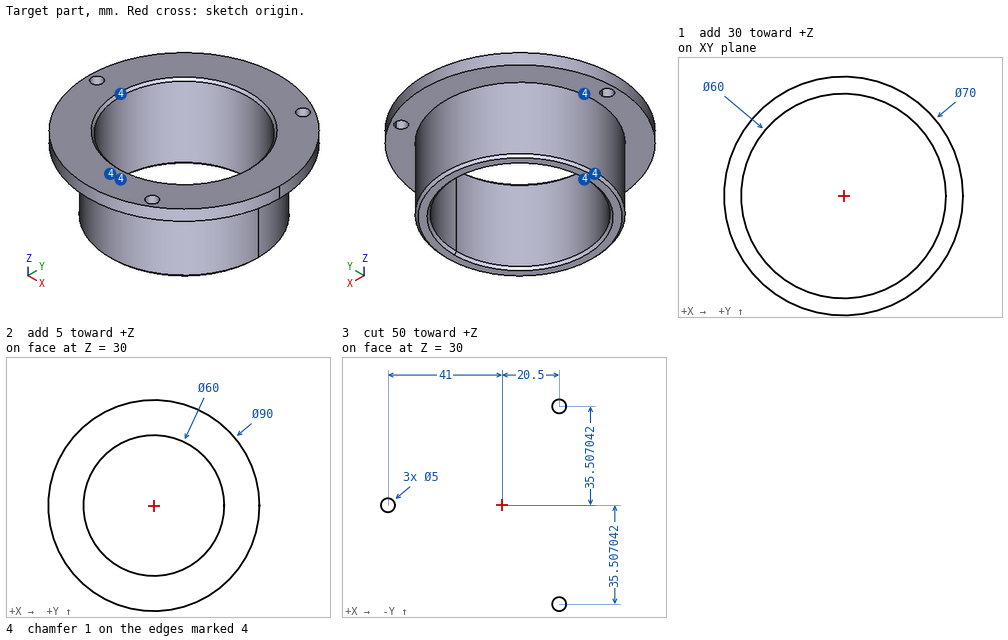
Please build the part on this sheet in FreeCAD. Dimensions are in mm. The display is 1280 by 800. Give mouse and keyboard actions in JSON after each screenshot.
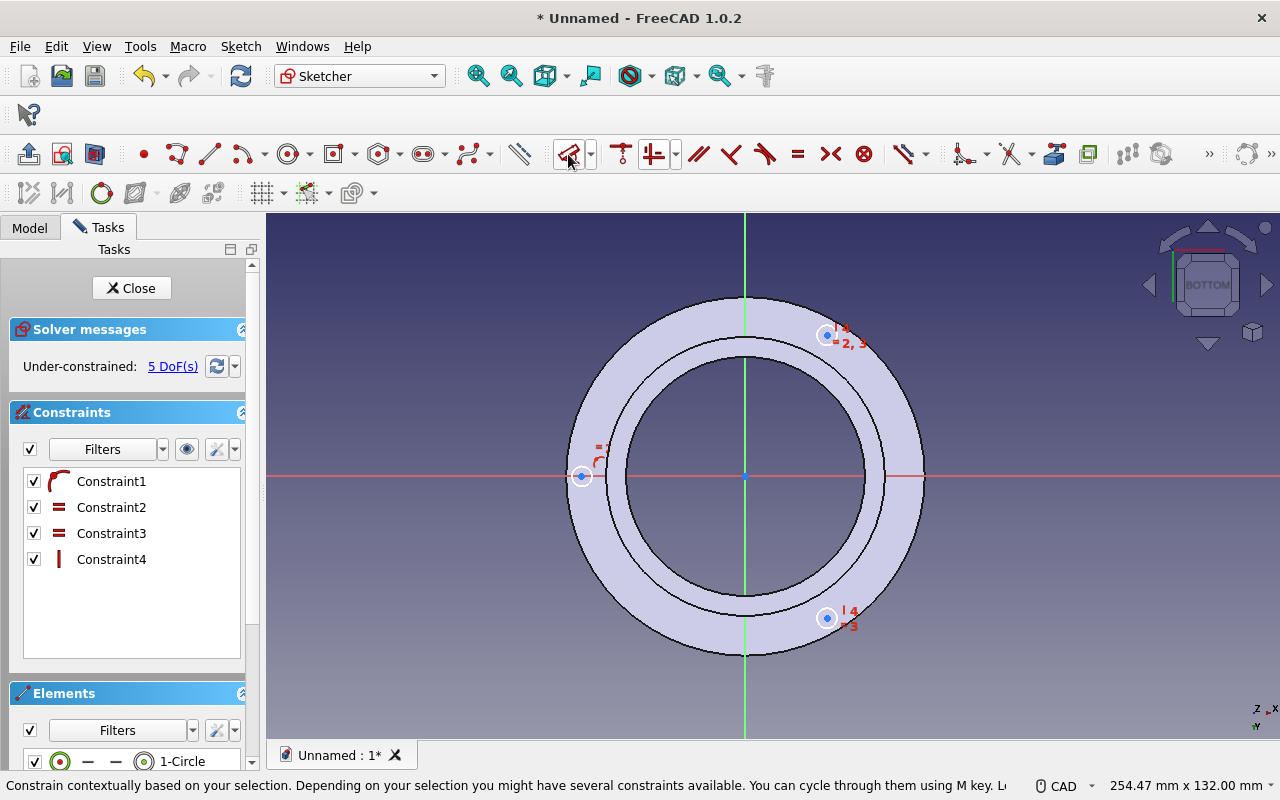
{"action": "scroll", "coordinate": [582, 466], "scroll_direction": "up", "scroll_amount": 4}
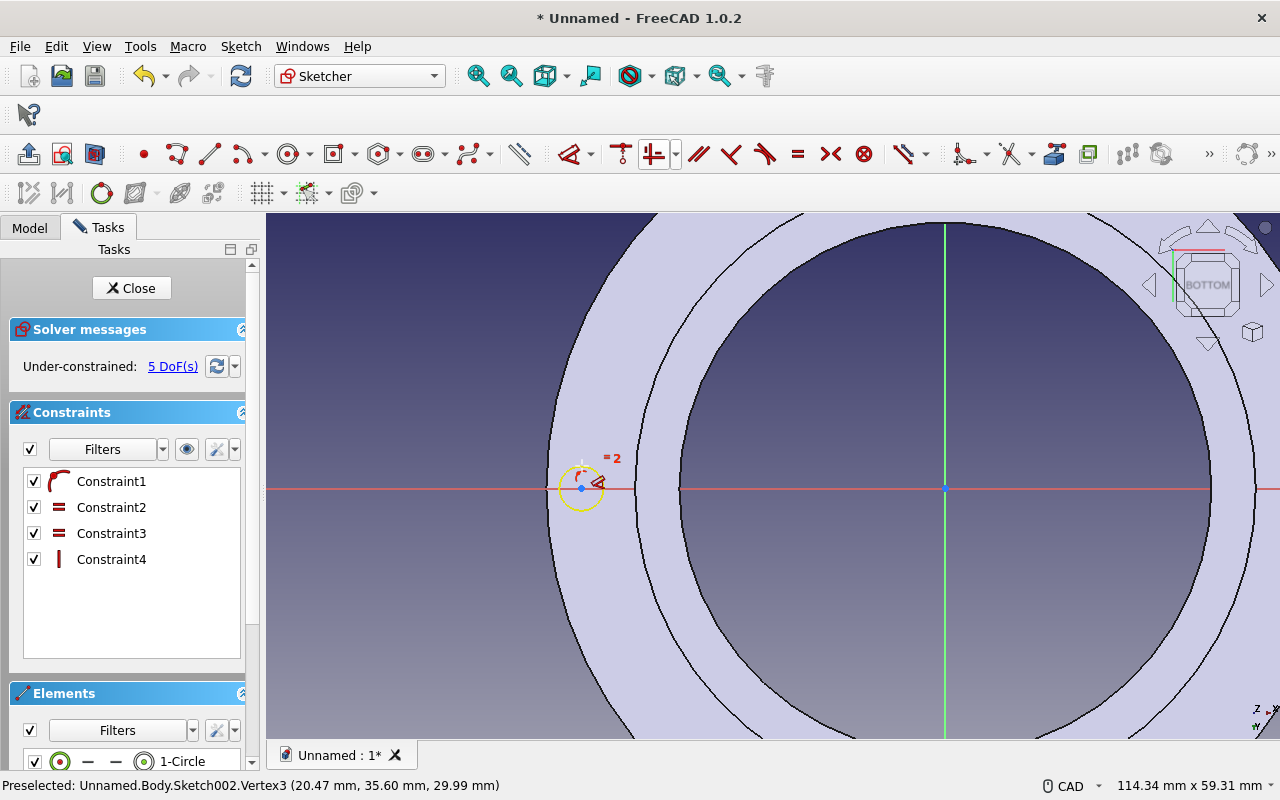
{"action": "left_click", "coordinate": [582, 466]}
{"action": "left_click", "coordinate": [583, 434]}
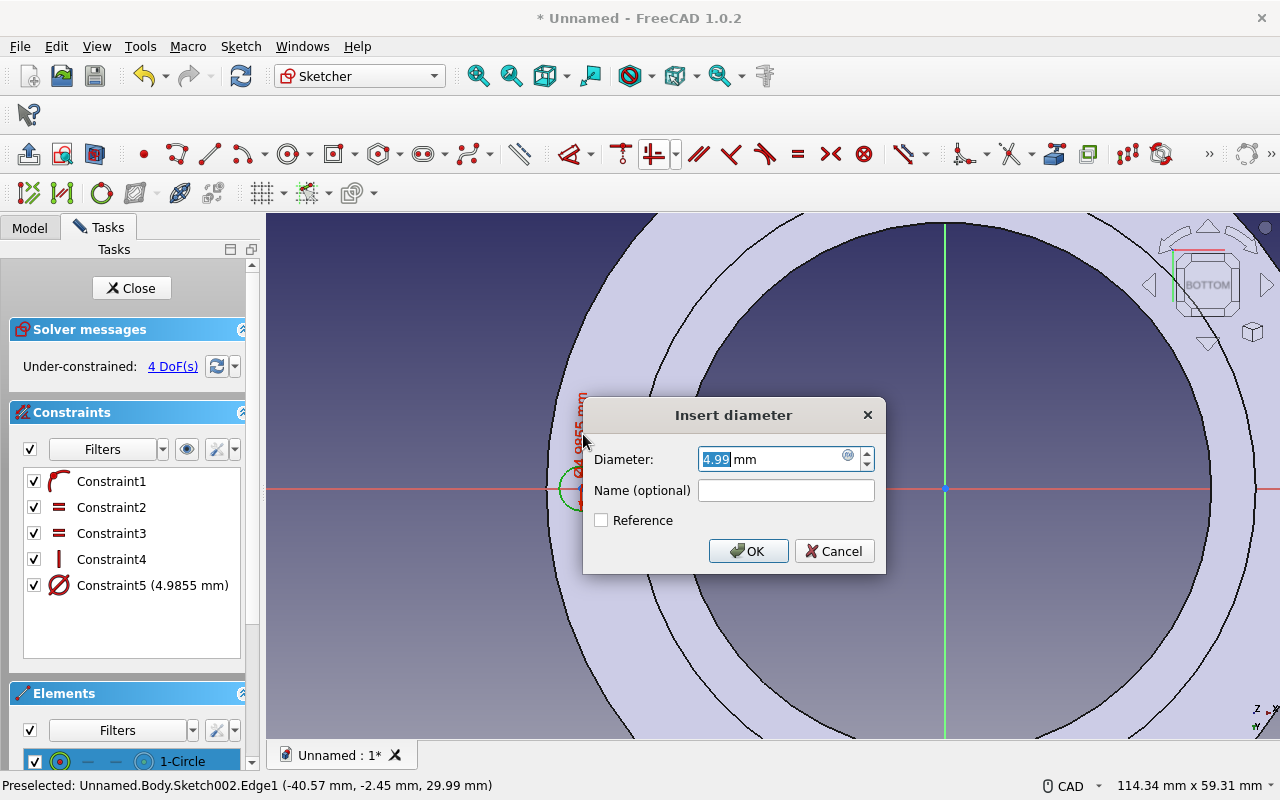
{"action": "type", "text": "5"}
{"action": "key", "text": "Return"}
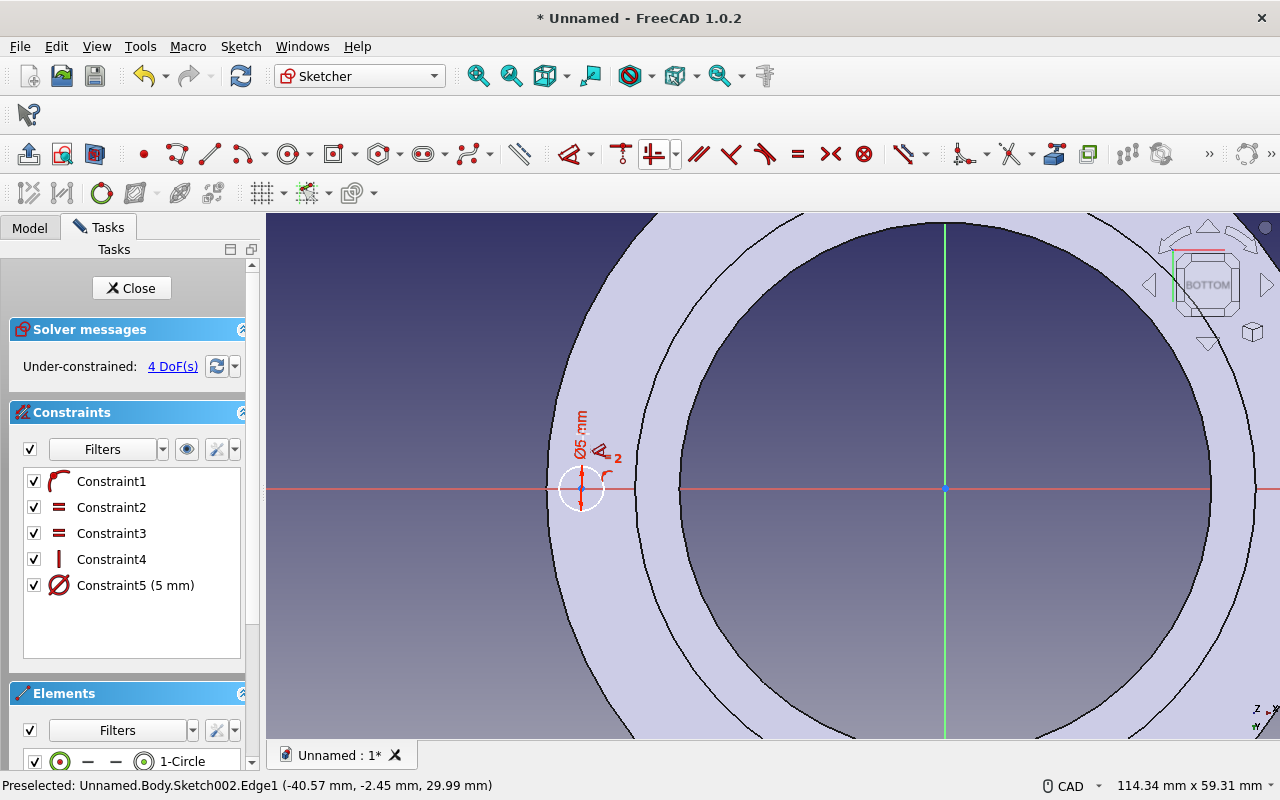
{"action": "left_click", "coordinate": [581, 489]}
{"action": "left_click", "coordinate": [763, 523]}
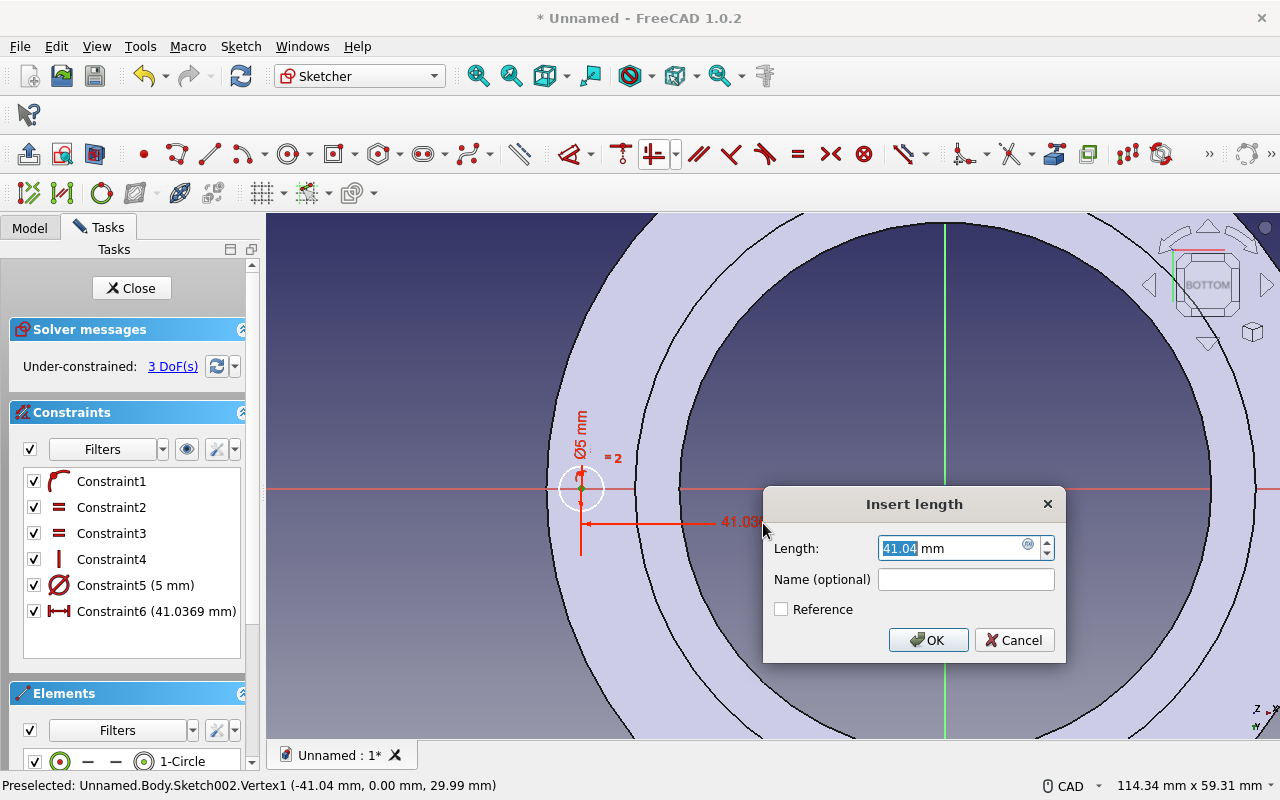
{"action": "type", "text": "41"}
{"action": "key", "text": "Return"}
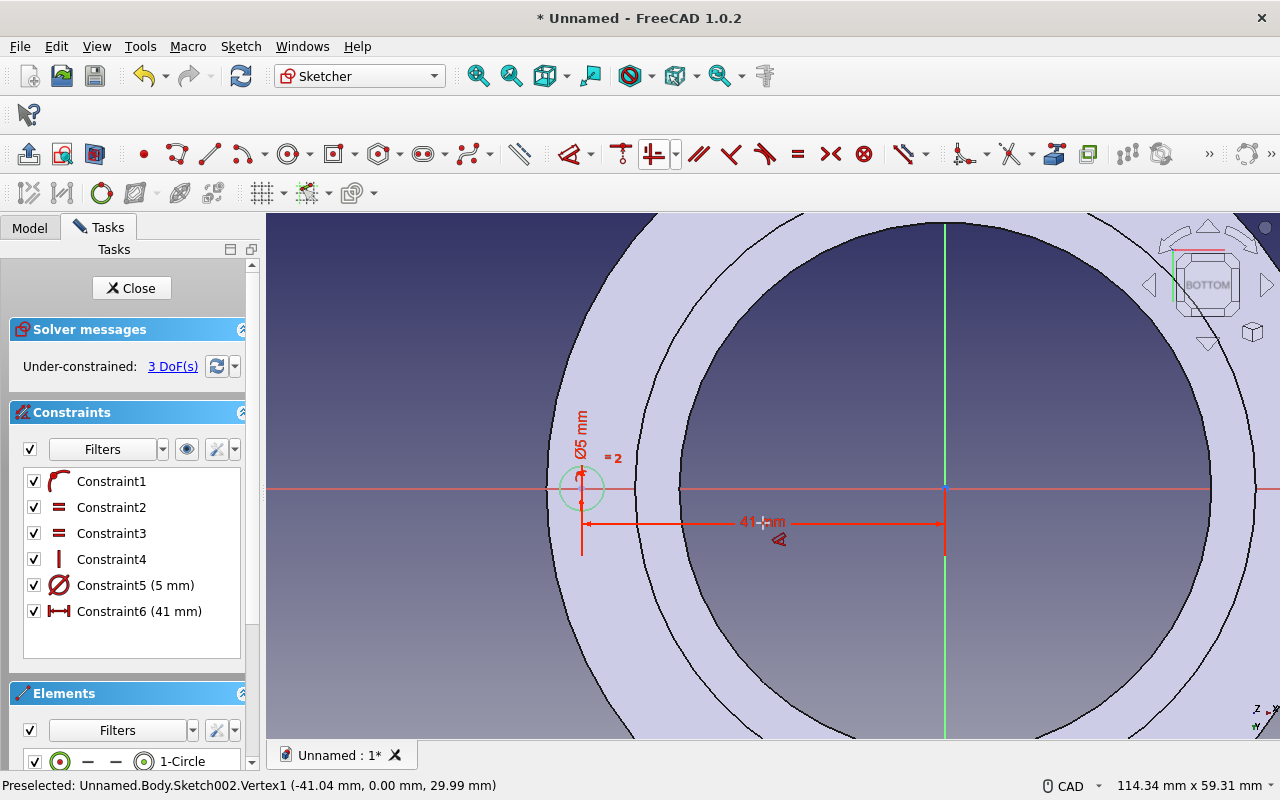
{"action": "scroll", "coordinate": [582, 466], "scroll_direction": "down", "scroll_amount": 4}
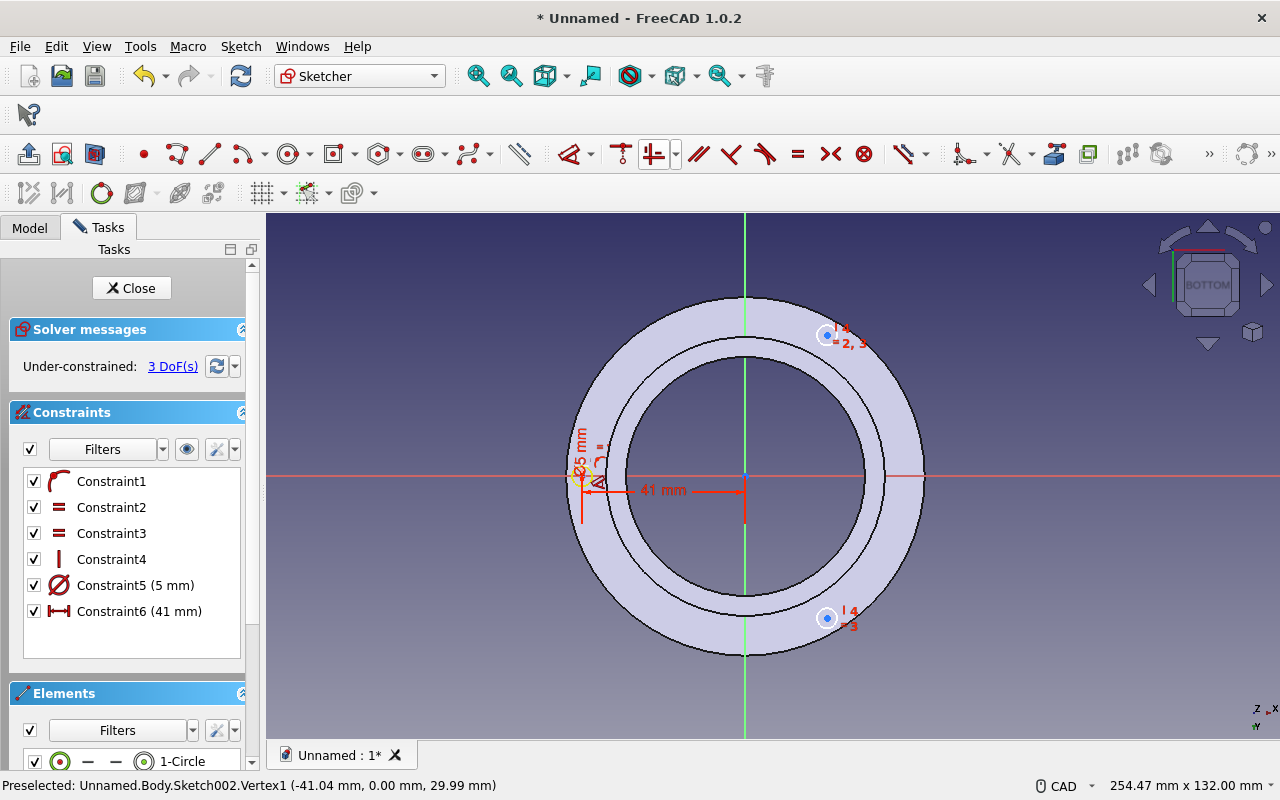
{"action": "left_click", "coordinate": [827, 335]}
{"action": "left_click", "coordinate": [786, 301]}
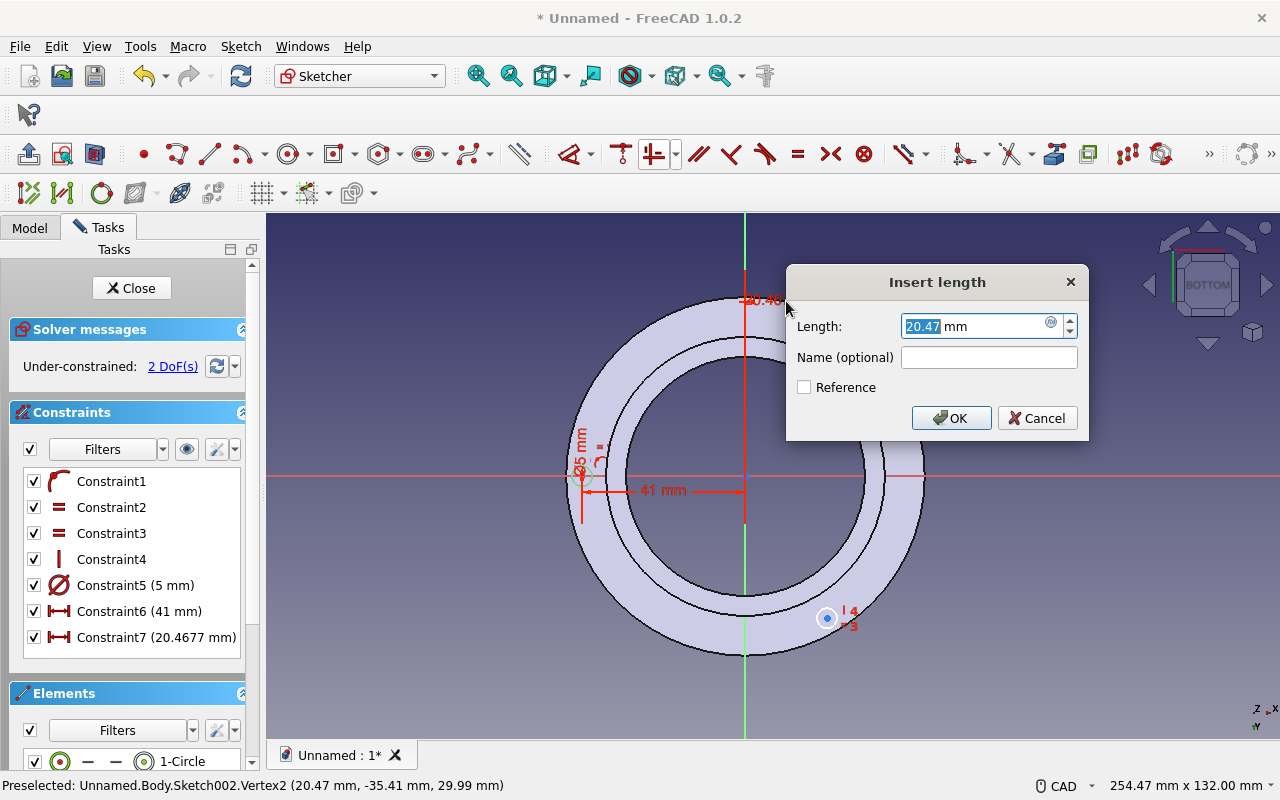
{"action": "type", "text": "20.5"}
{"action": "key", "text": "Return"}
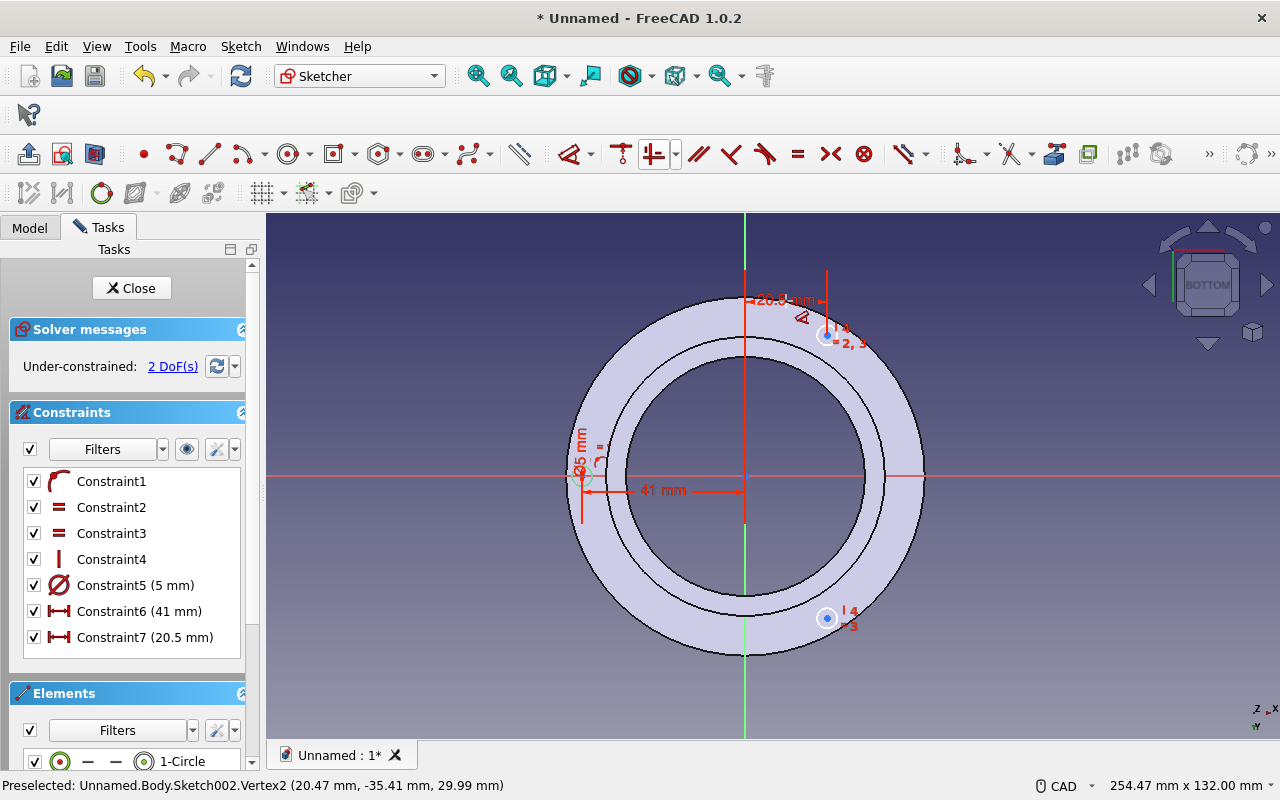
{"action": "left_click", "coordinate": [827, 335]}
{"action": "left_click", "coordinate": [861, 406]}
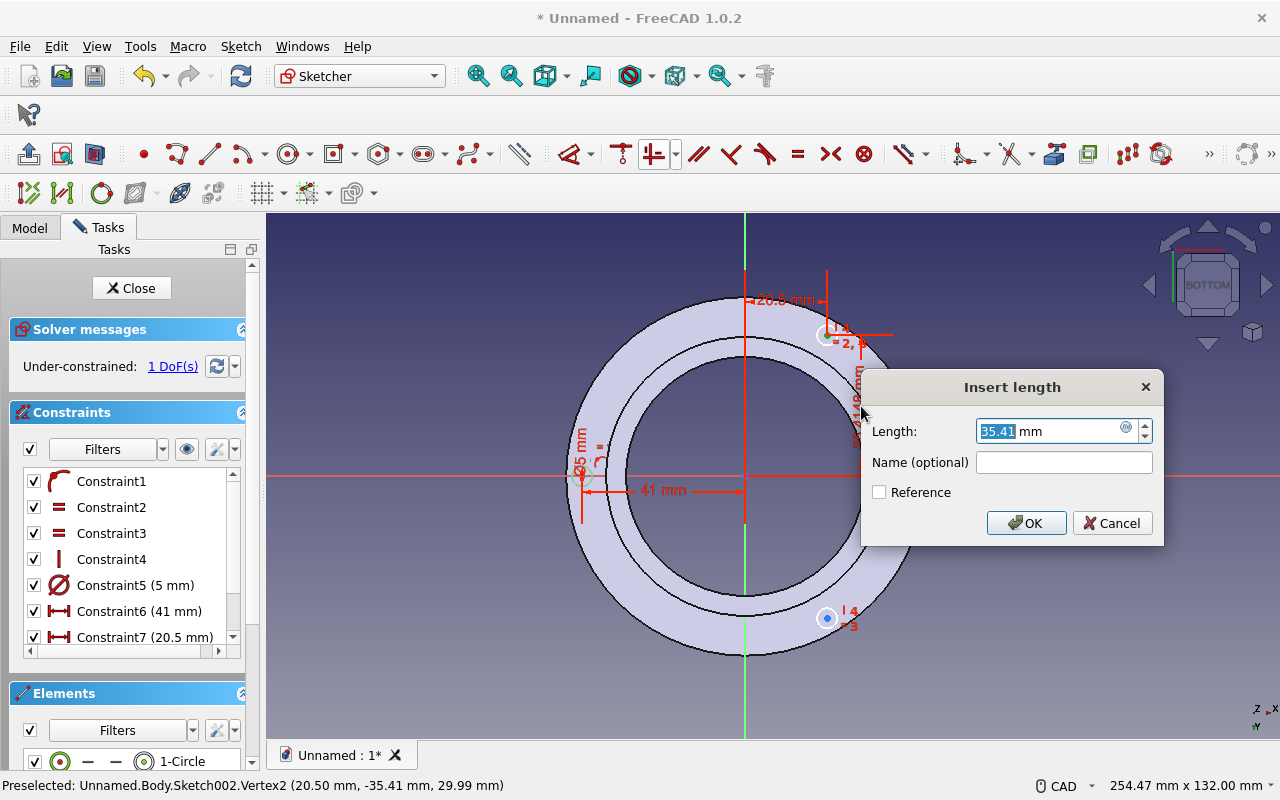
{"action": "type", "text": "35.507042"}
{"action": "key", "text": "Return"}